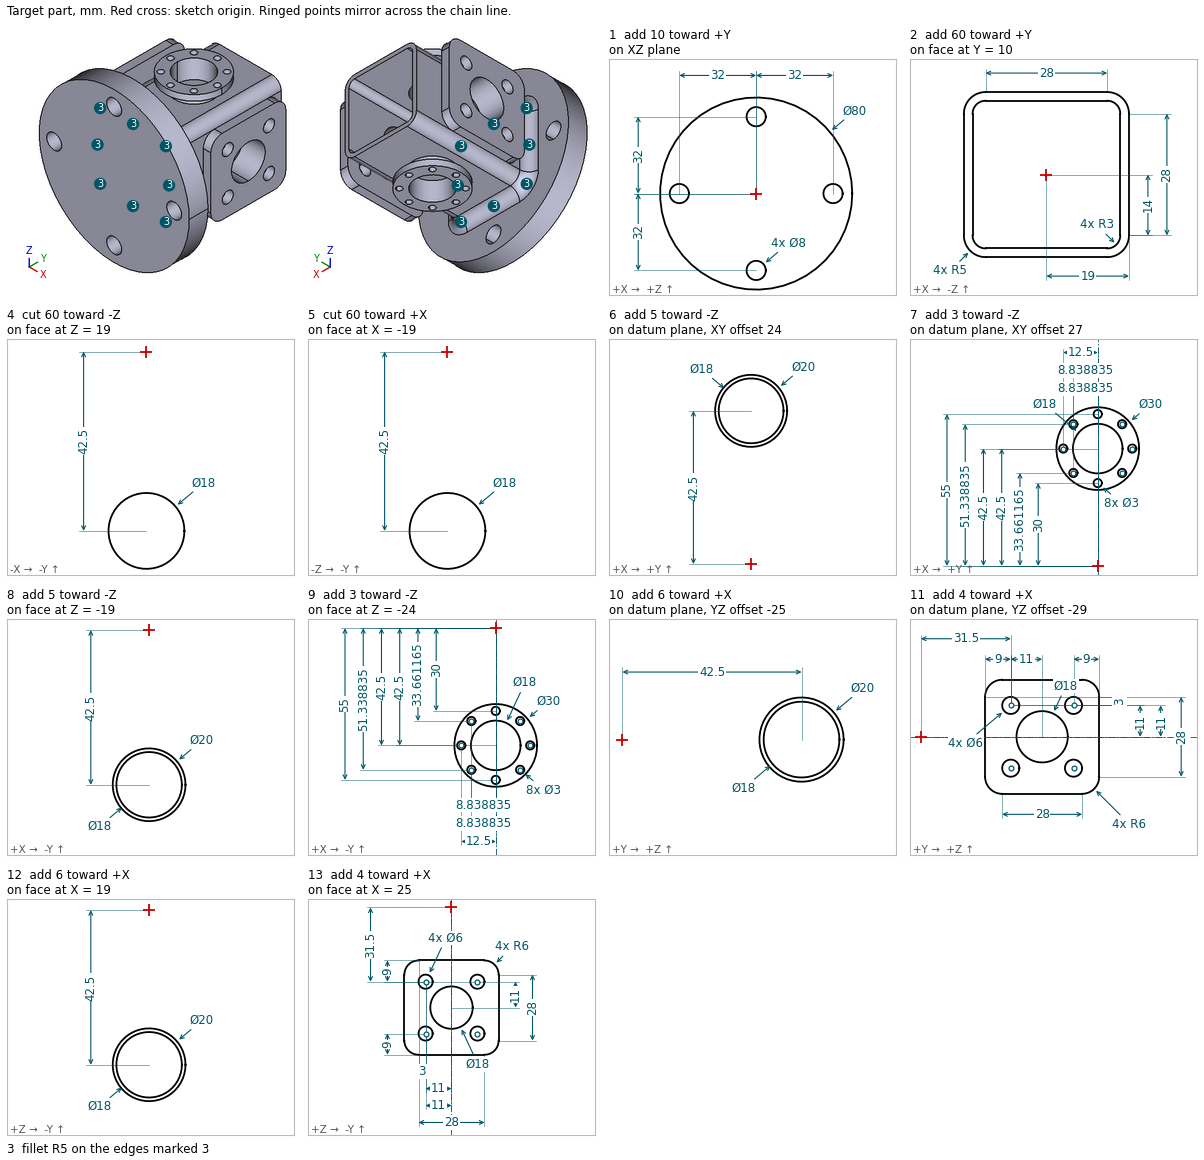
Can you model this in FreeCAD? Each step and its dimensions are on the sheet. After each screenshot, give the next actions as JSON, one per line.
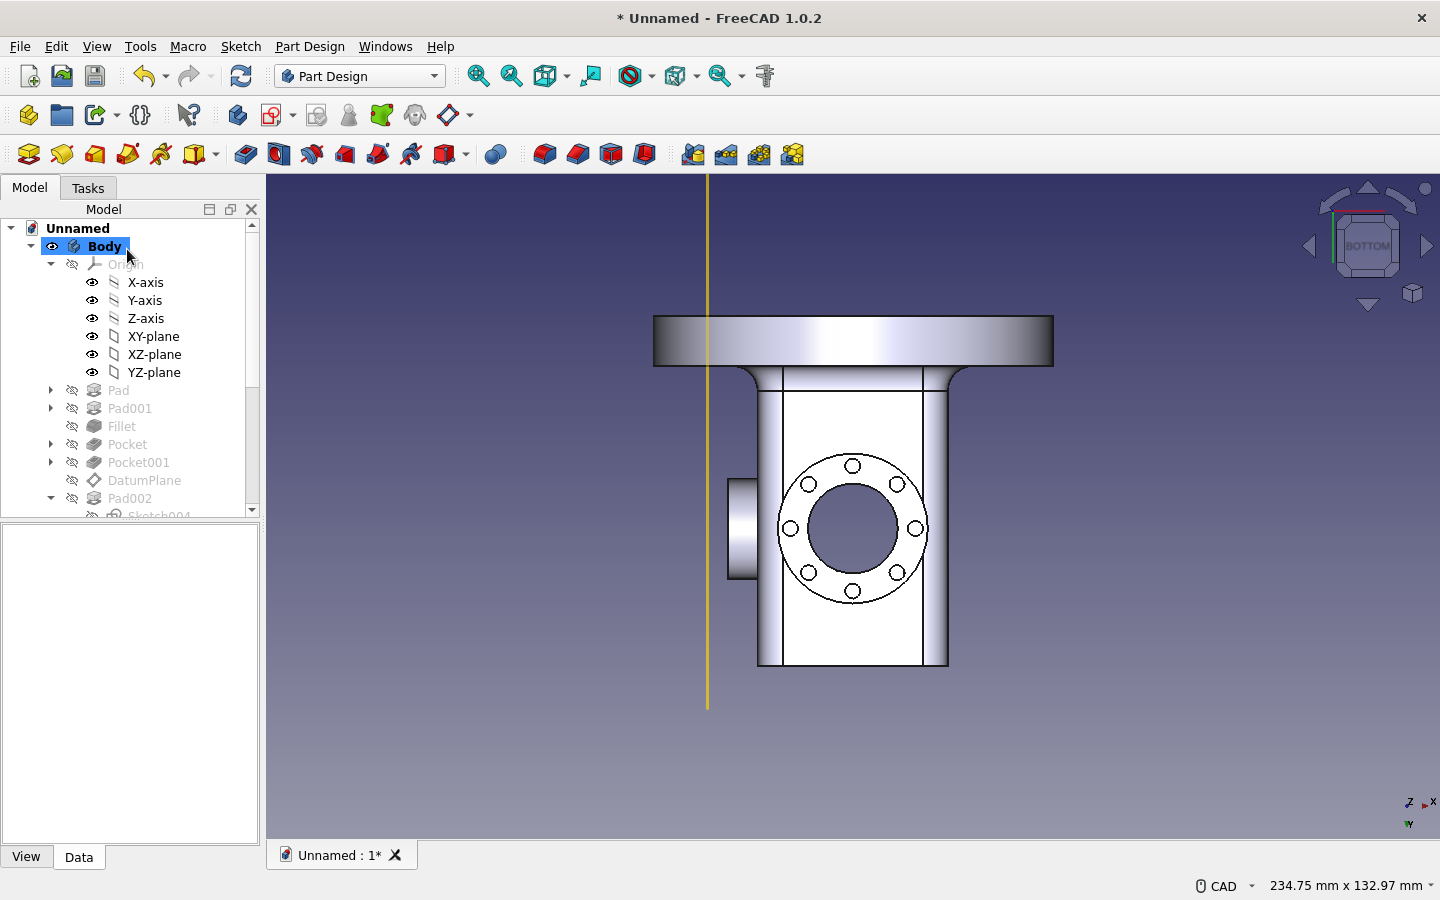
{"action": "scroll", "coordinate": [101, 368], "scroll_direction": "down", "scroll_amount": 3}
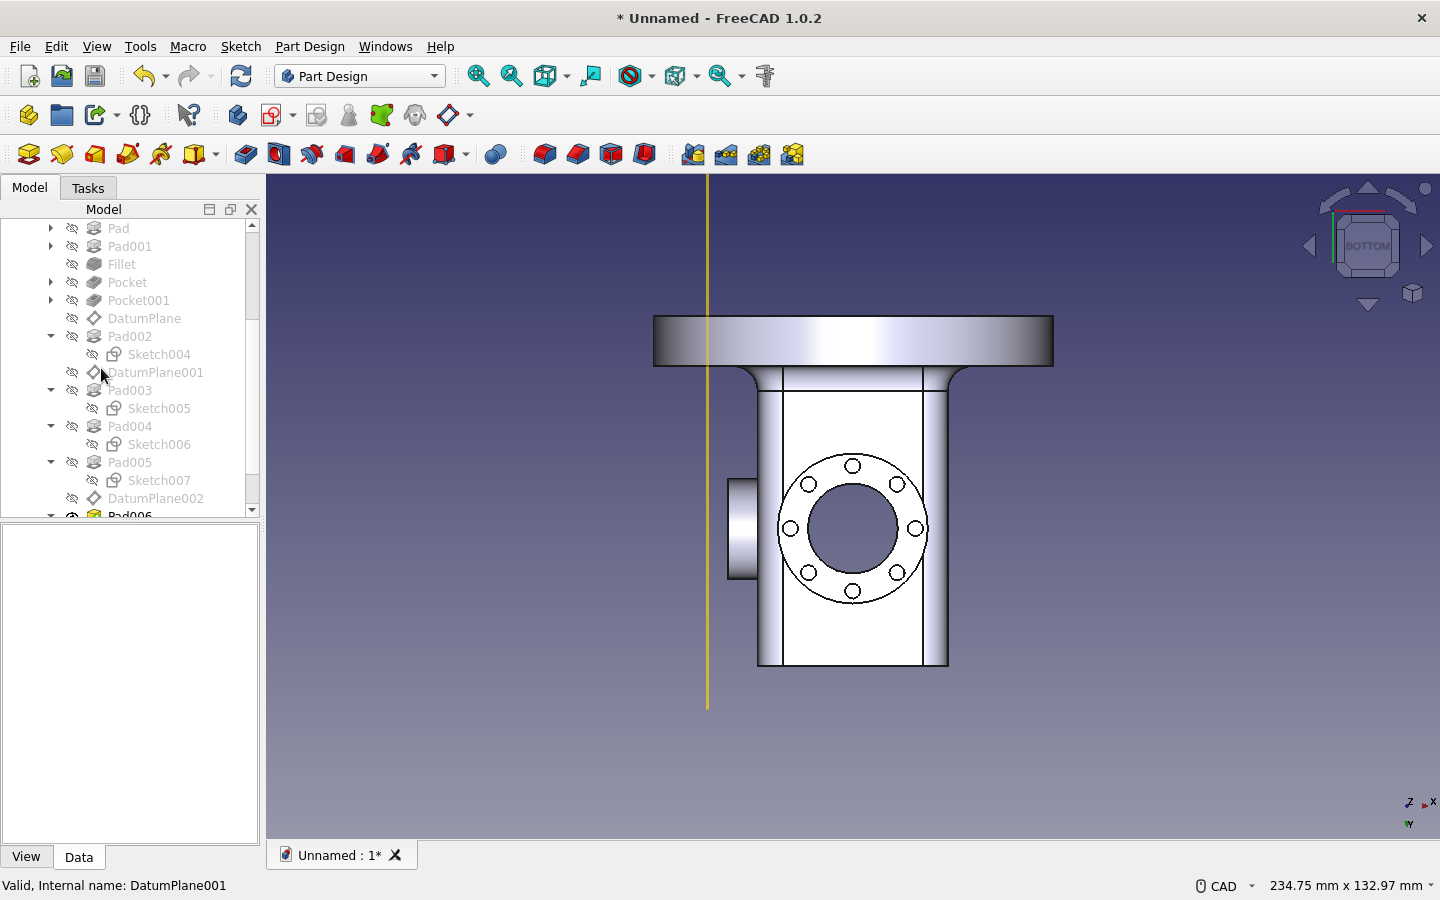
{"action": "scroll", "coordinate": [141, 368], "scroll_direction": "up", "scroll_amount": 15}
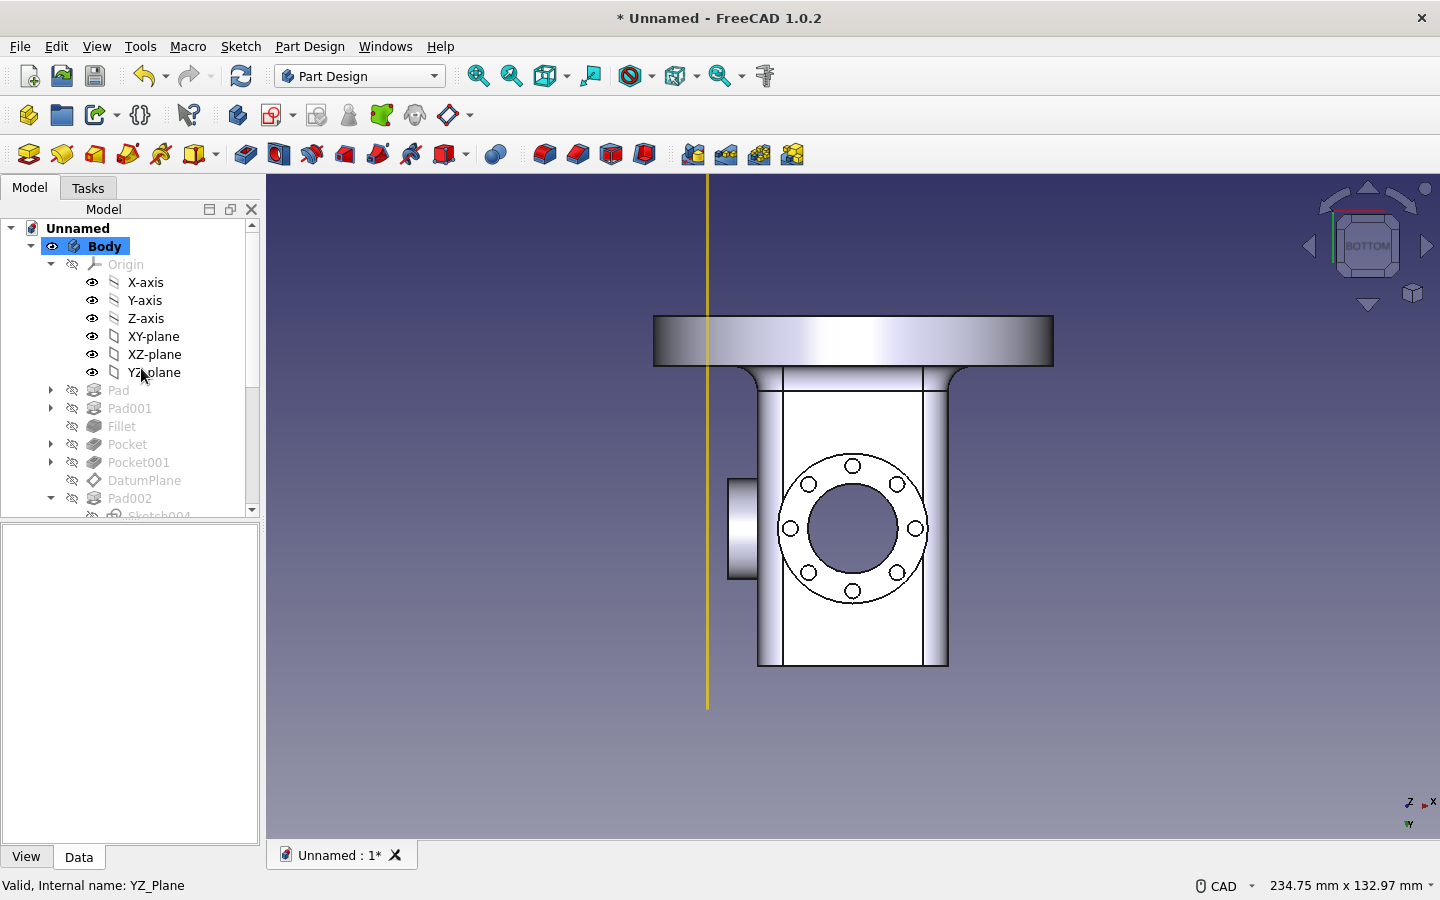
{"action": "scroll", "coordinate": [101, 368], "scroll_direction": "down", "scroll_amount": 6}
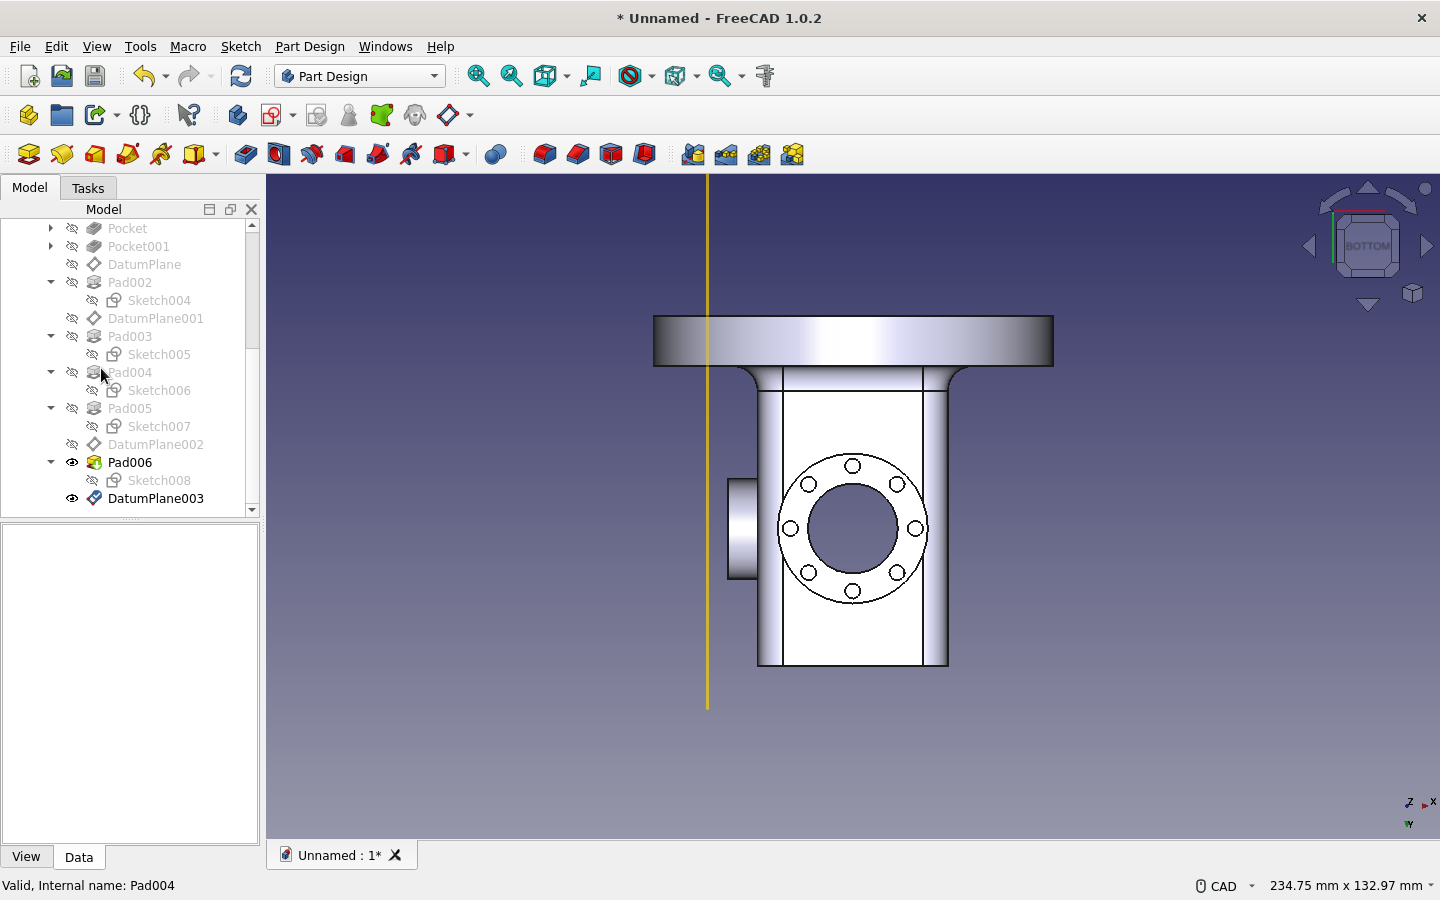
{"action": "left_click", "coordinate": [117, 498]}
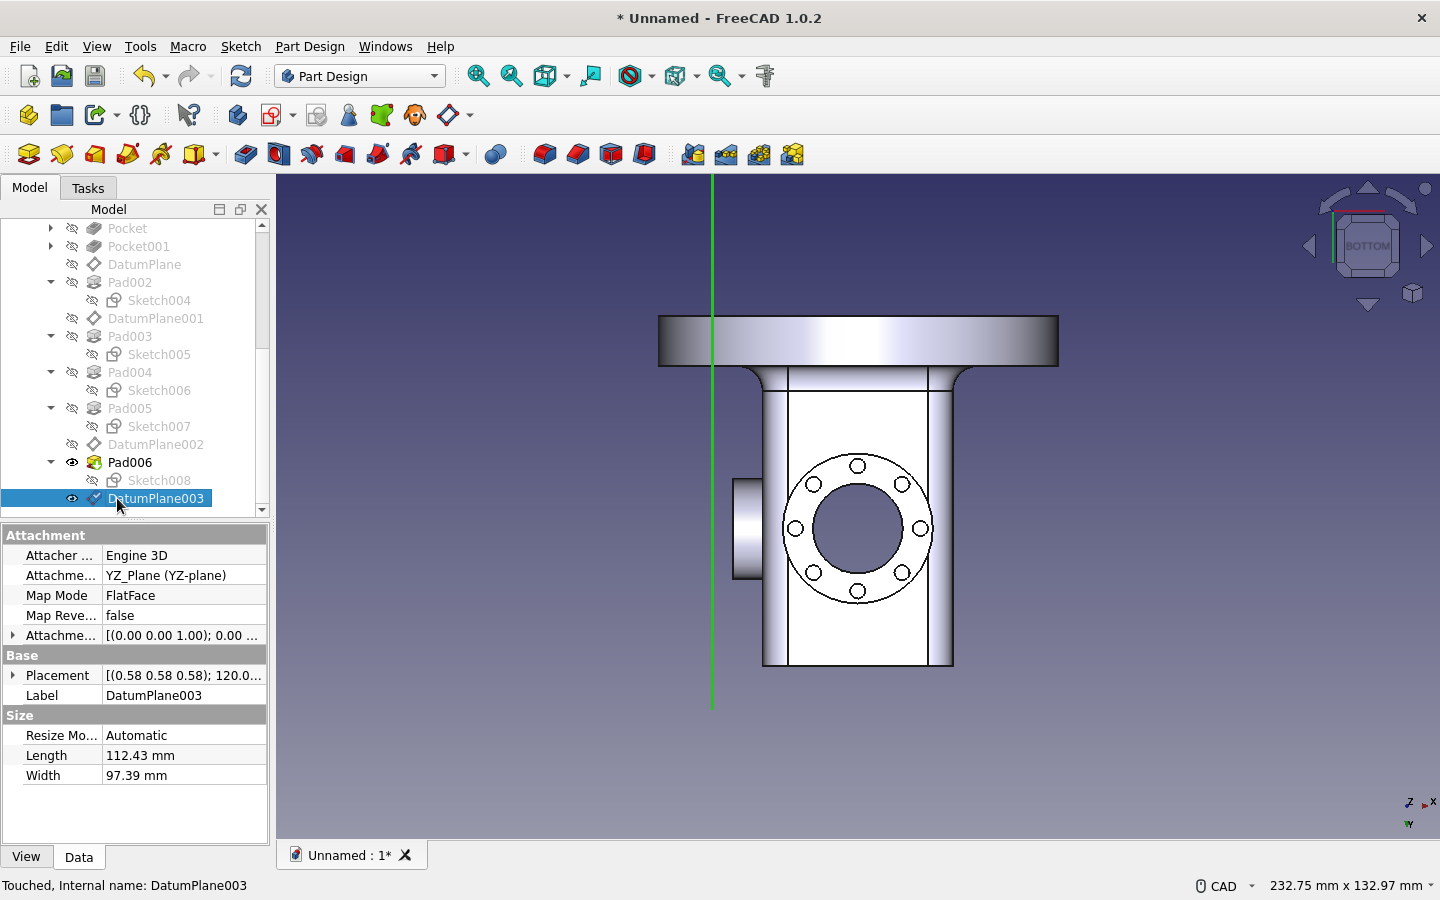
{"action": "left_click", "coordinate": [270, 116]}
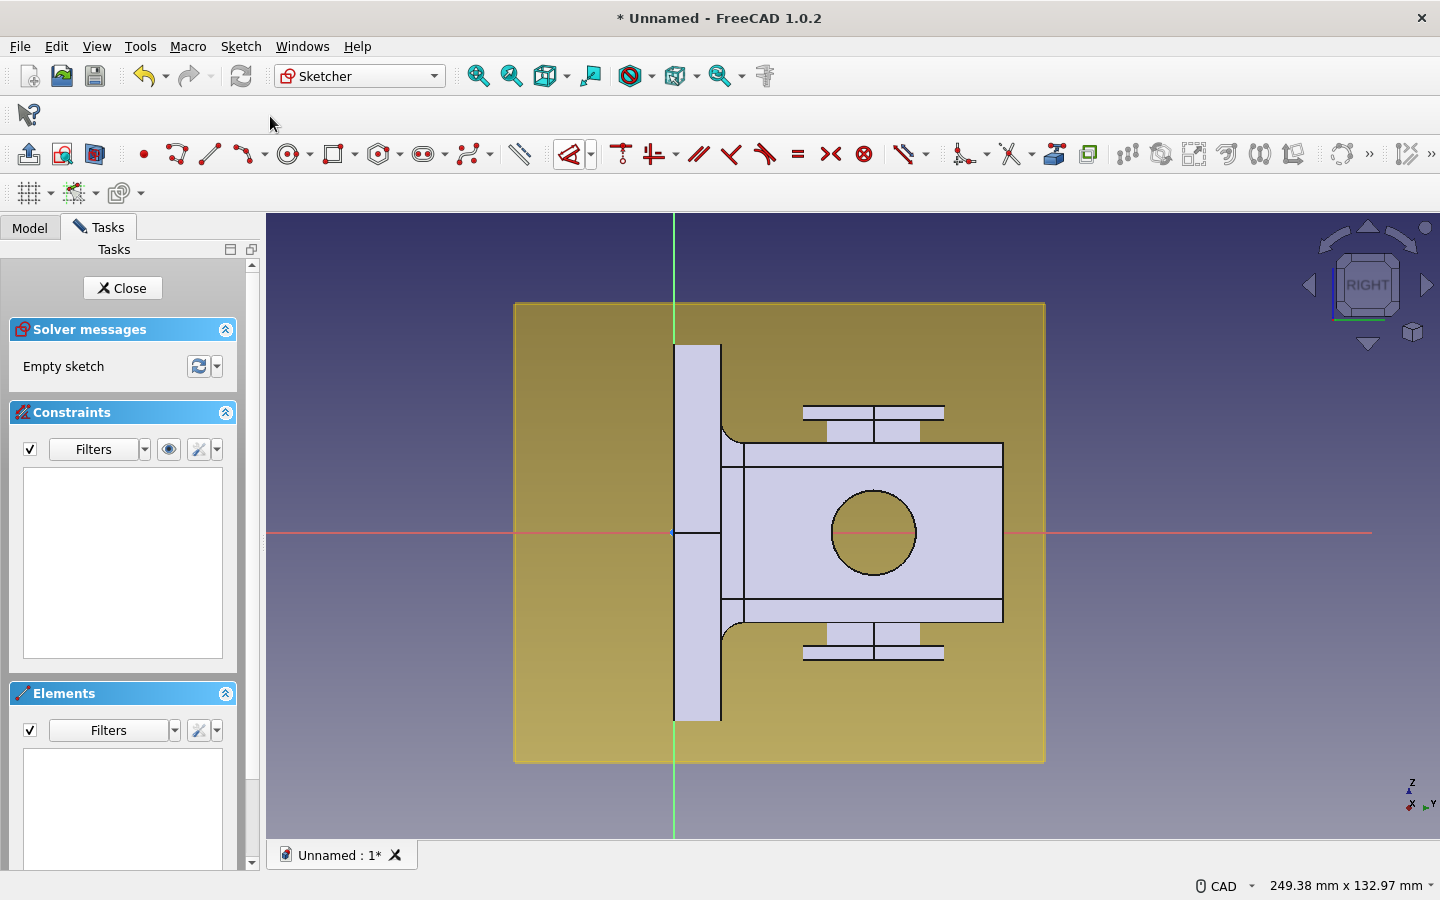
{"action": "key", "text": "q s"}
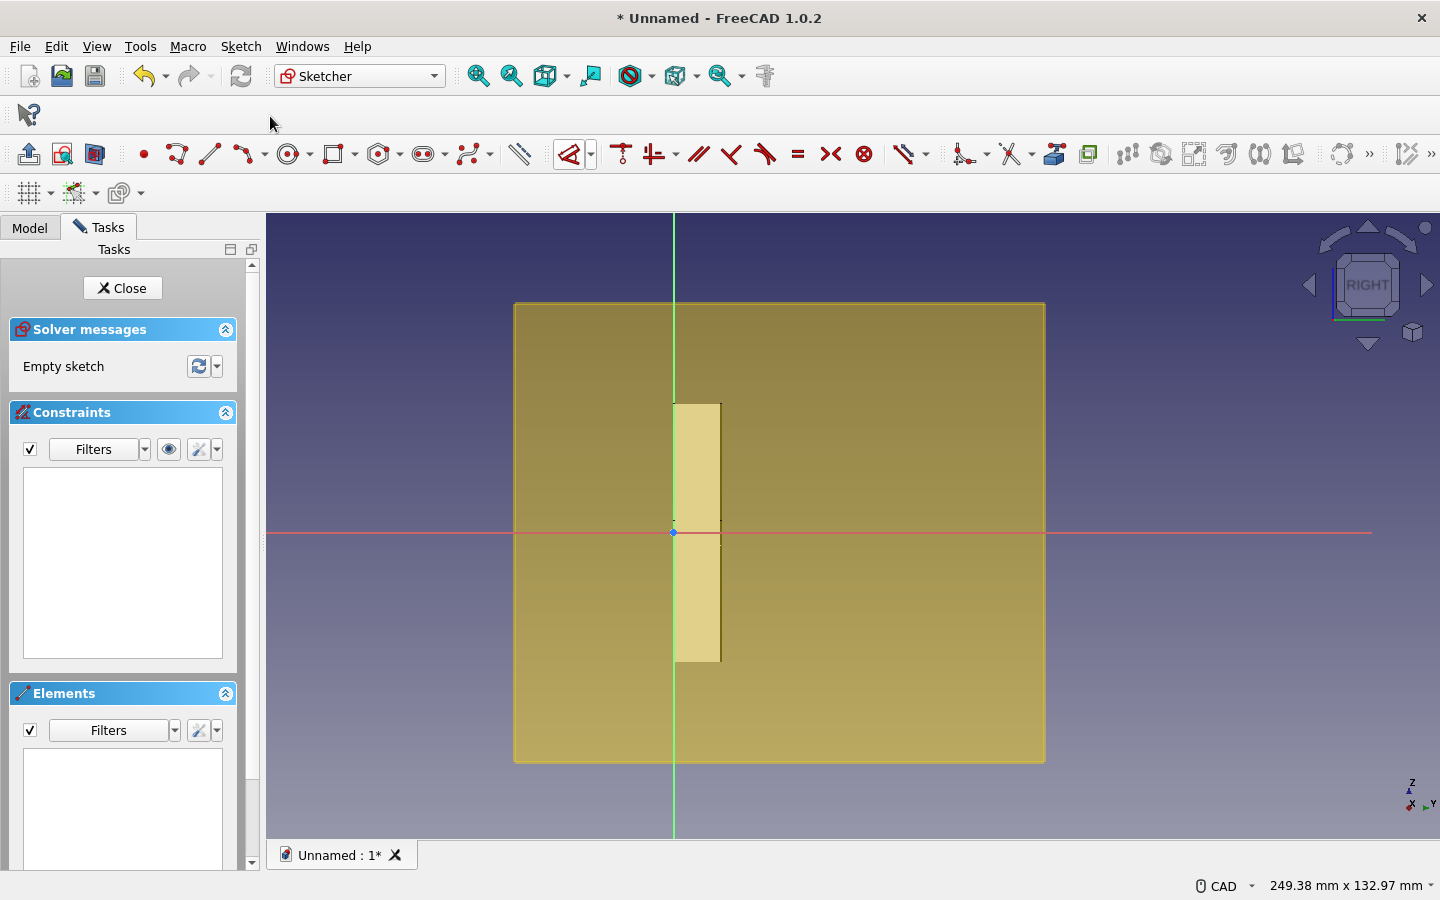
{"action": "scroll", "coordinate": [850, 538], "scroll_direction": "up", "scroll_amount": 4}